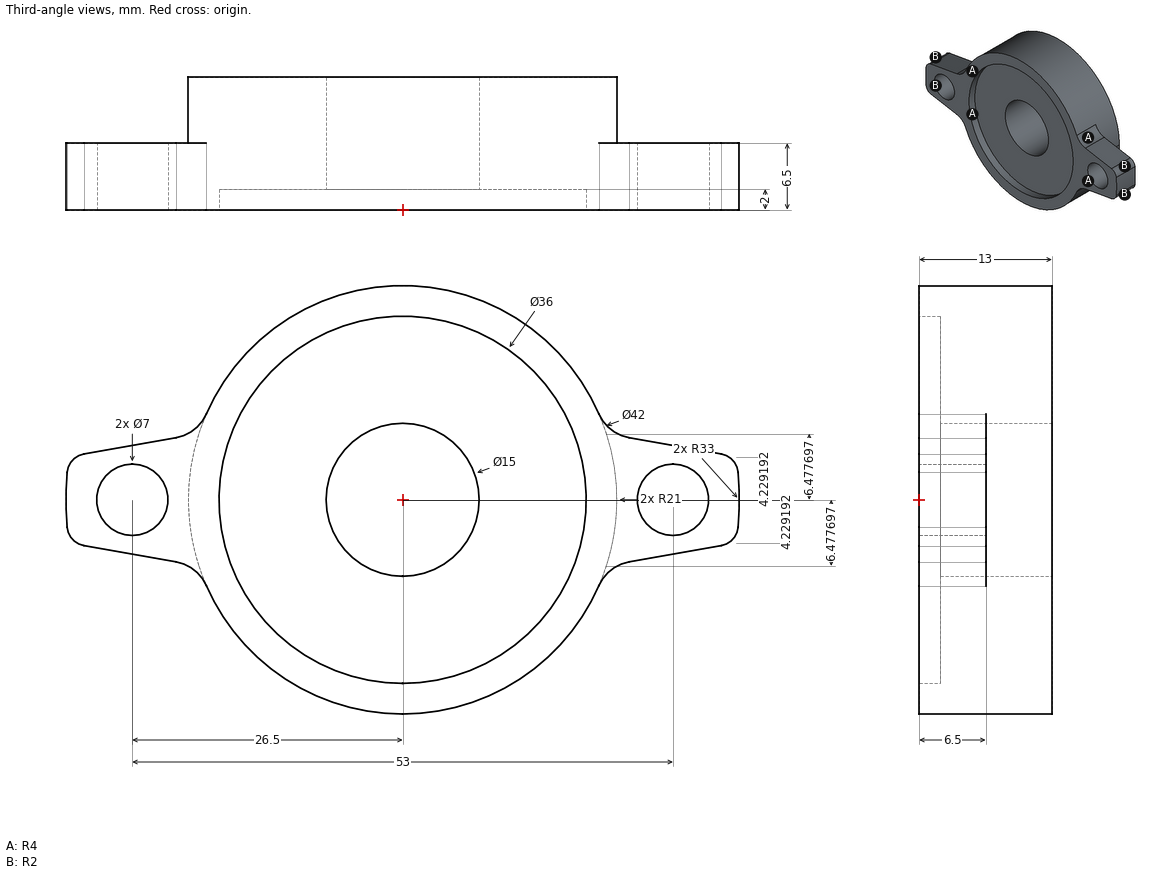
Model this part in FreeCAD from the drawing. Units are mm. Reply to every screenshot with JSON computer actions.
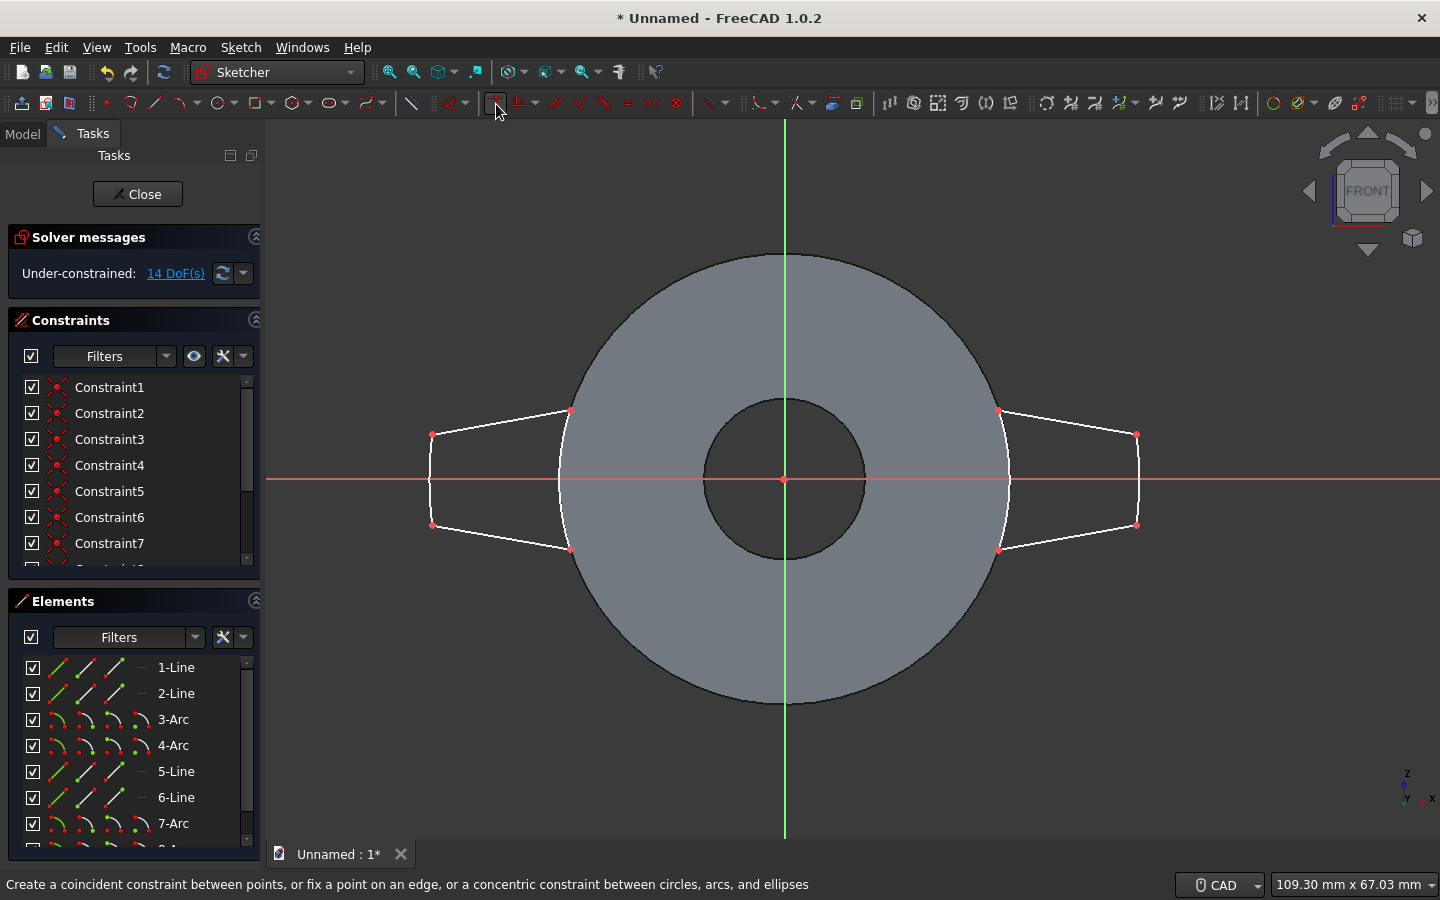
{"action": "left_click_drag", "start_coordinate": [774, 469], "coordinate": [795, 490]}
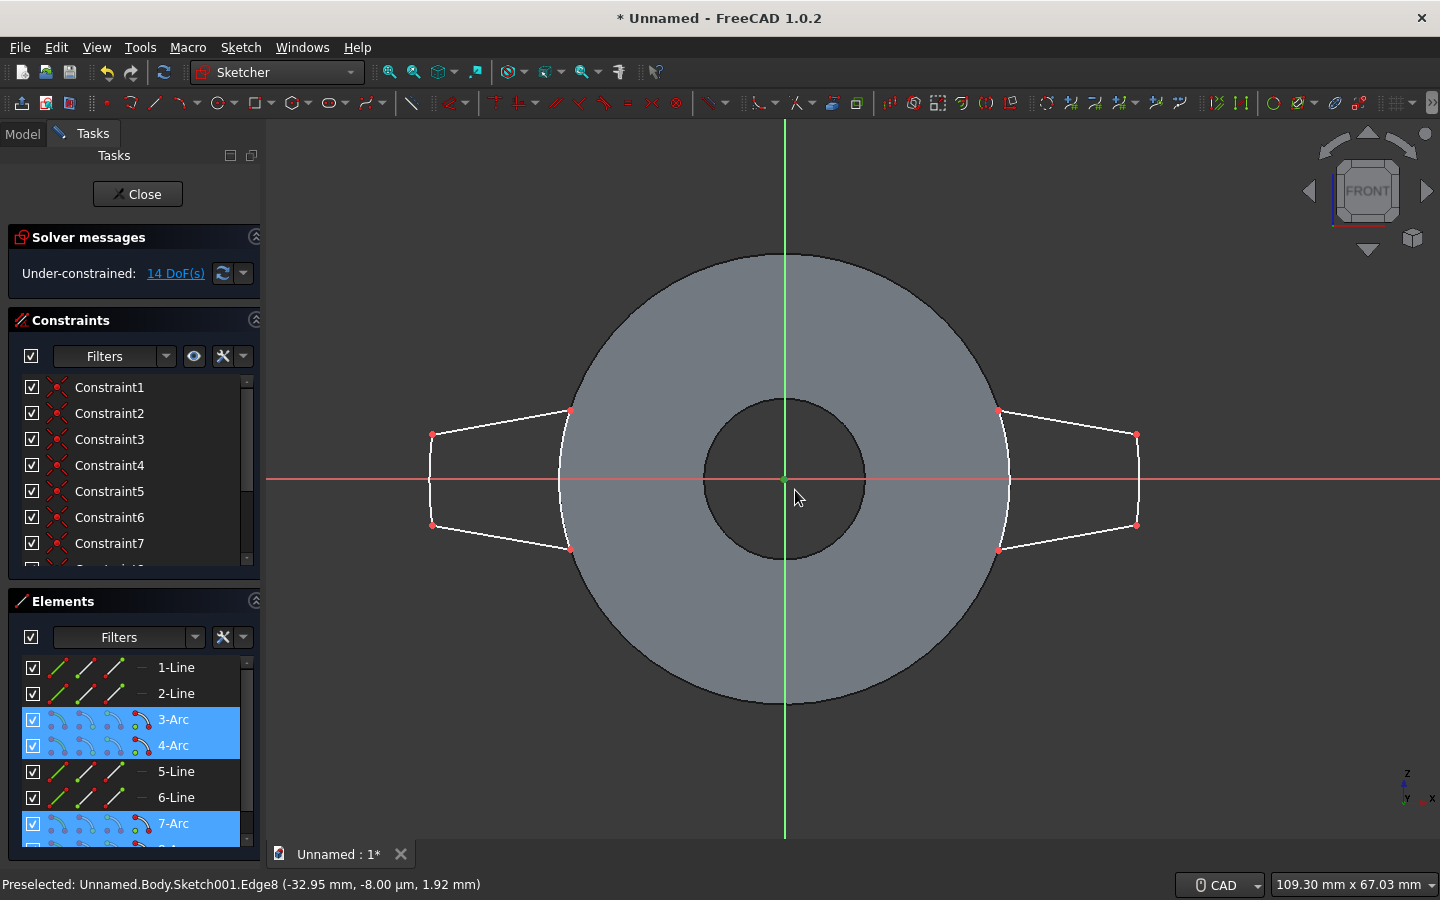
{"action": "left_click", "coordinate": [496, 104]}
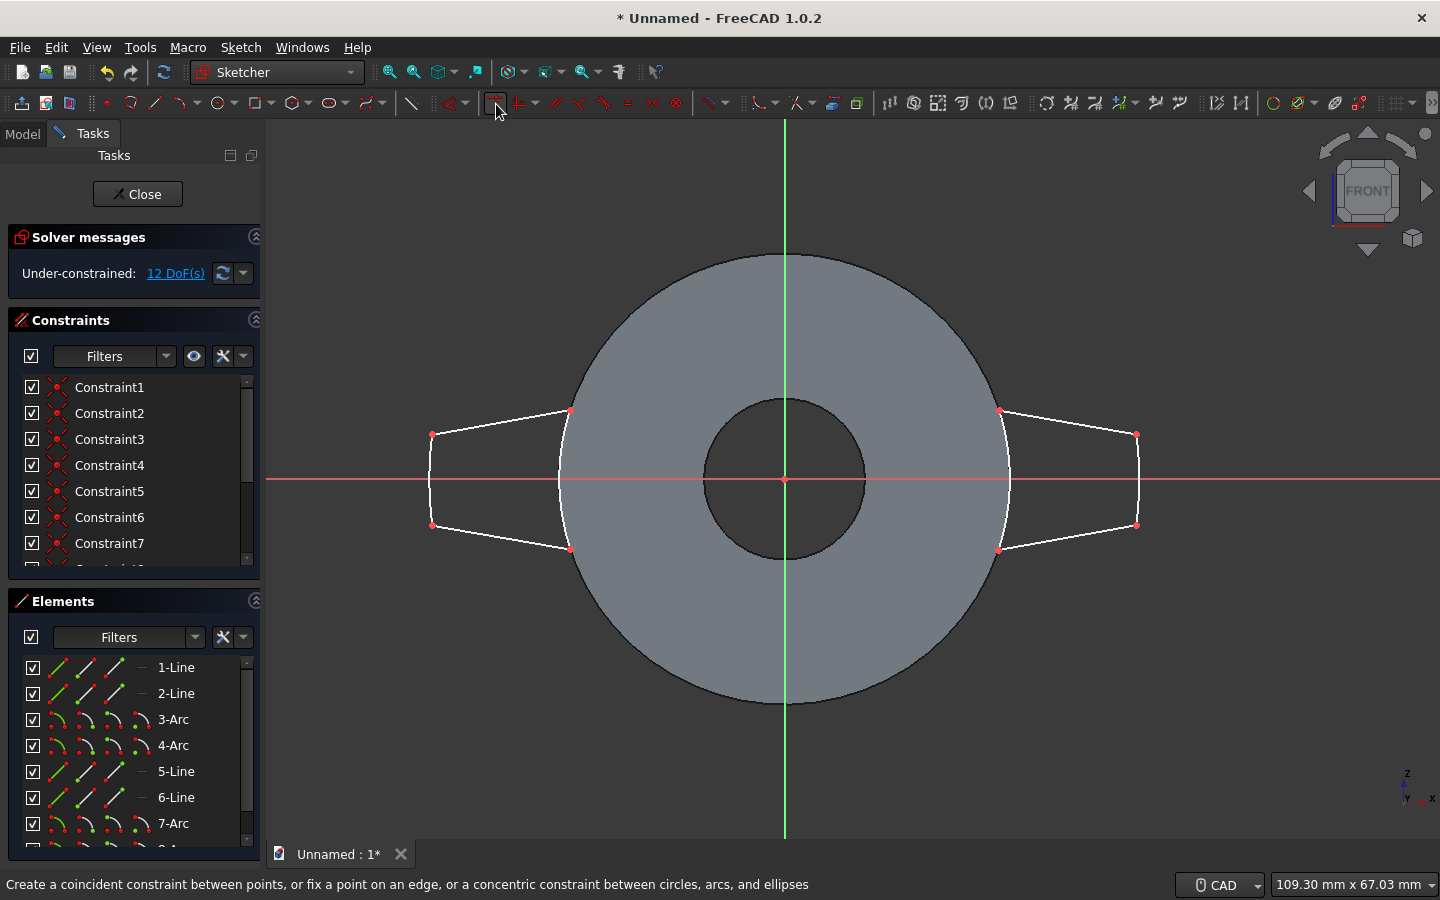
{"action": "left_click", "coordinate": [1008, 509]}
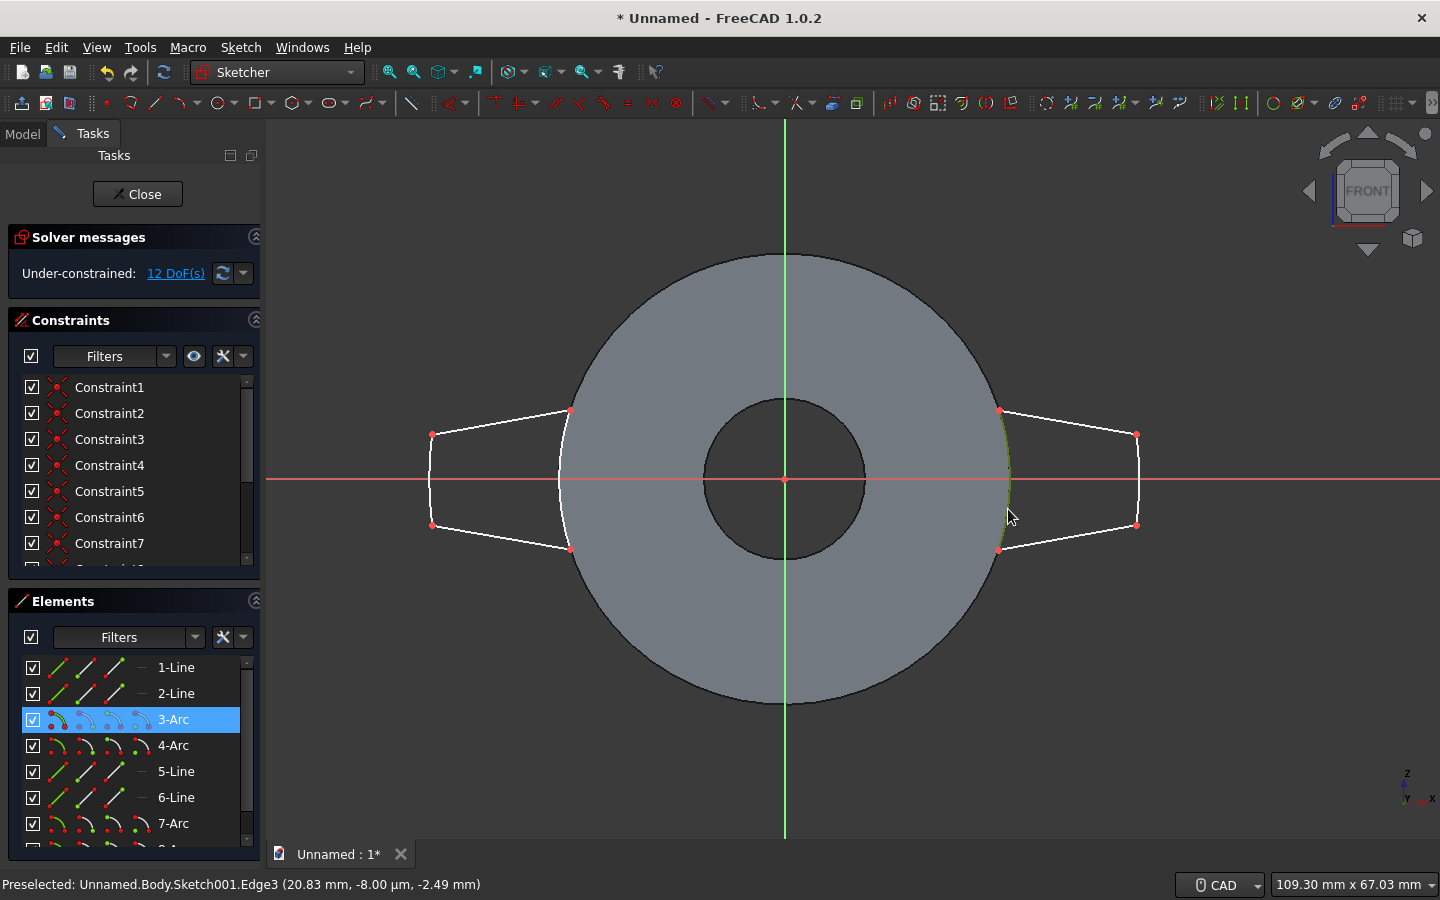
{"action": "left_click", "coordinate": [561, 452]}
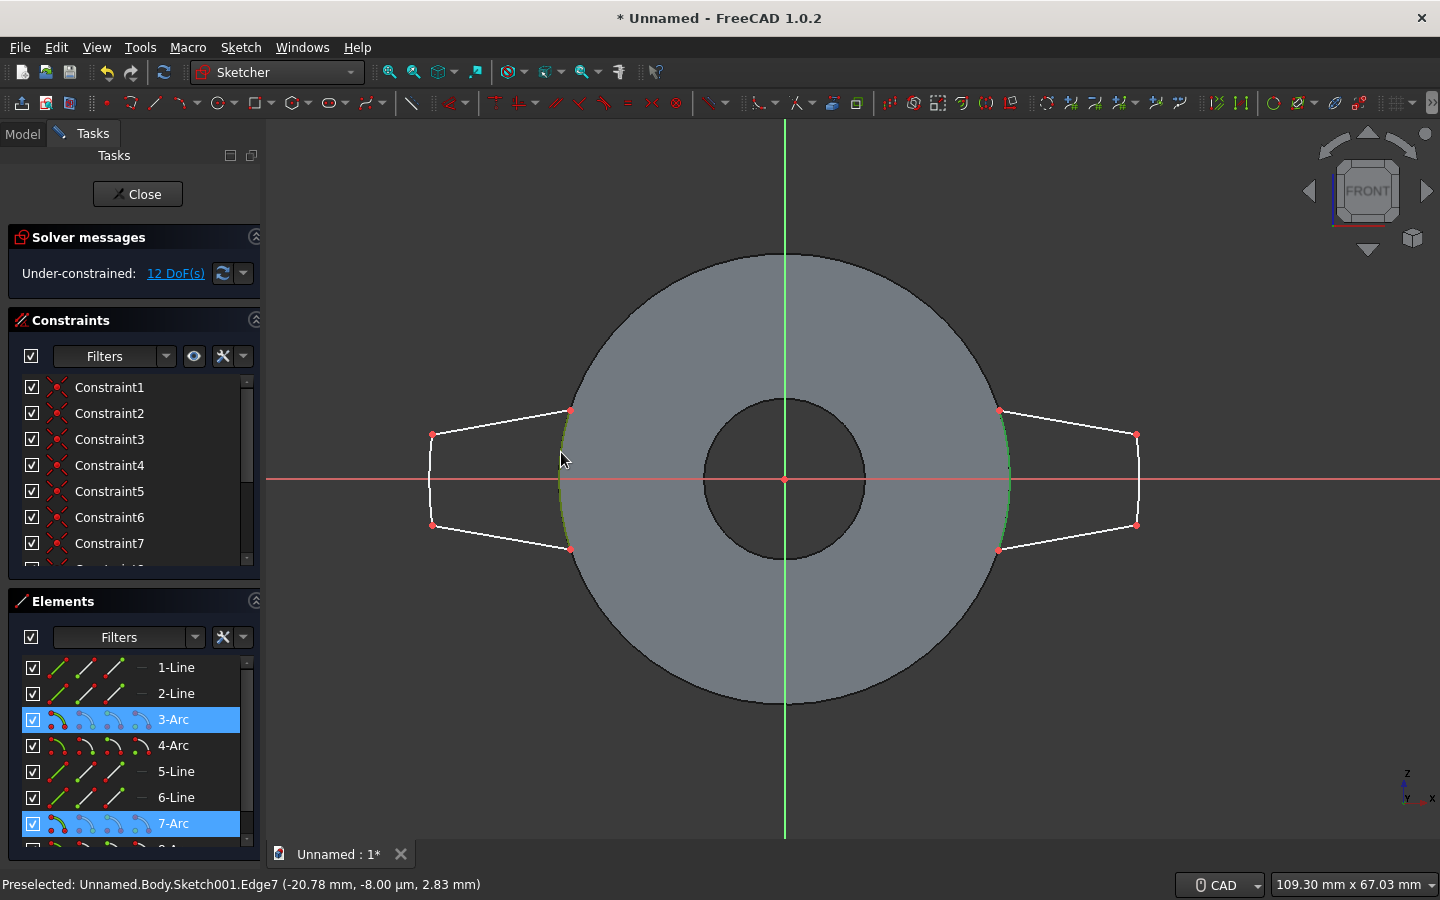
{"action": "left_click", "coordinate": [628, 104]}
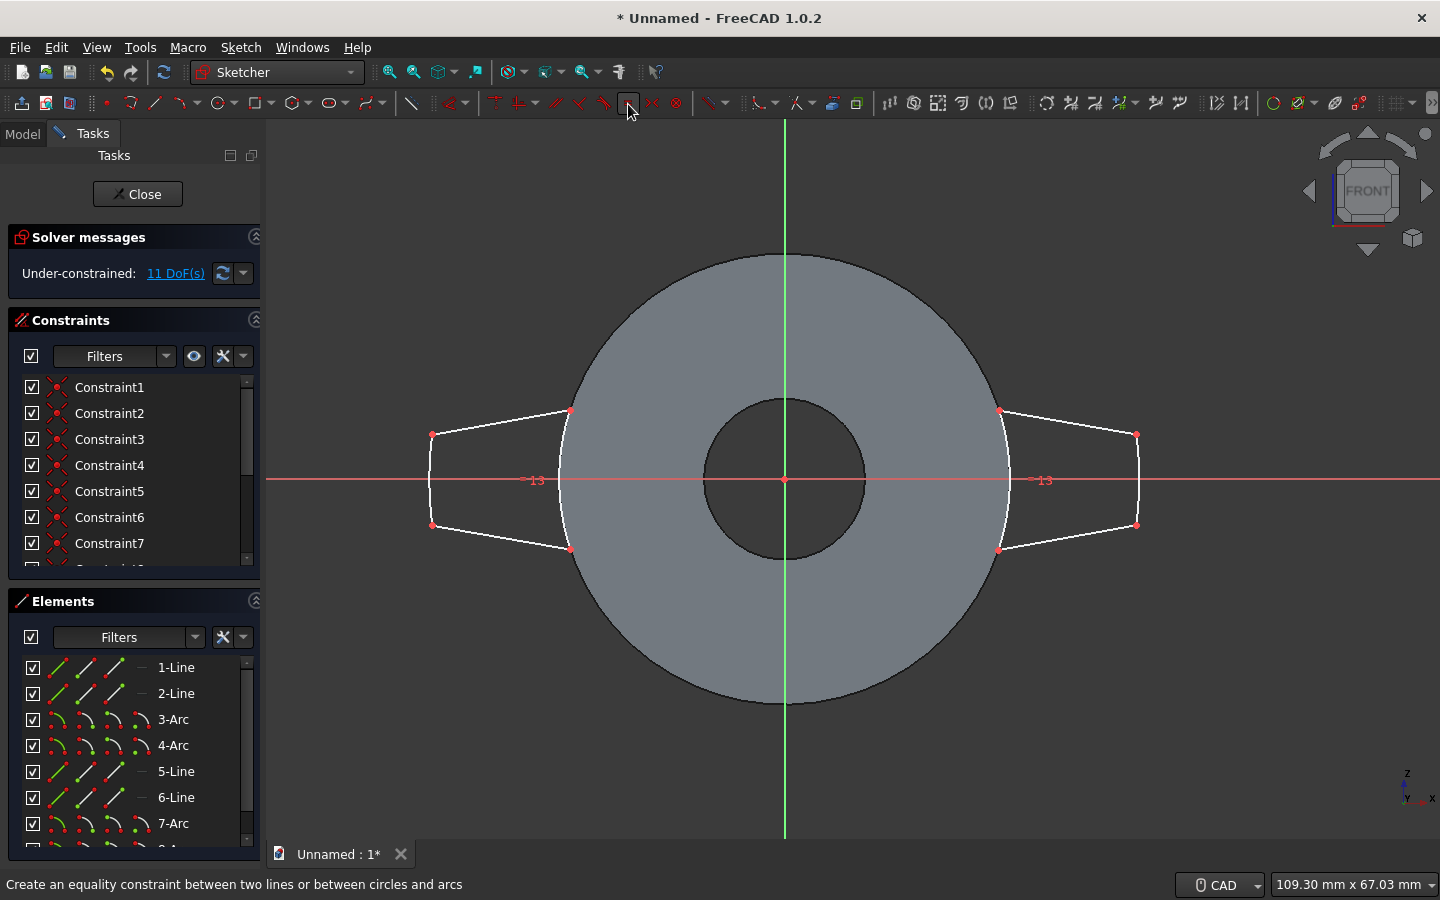
{"action": "left_click", "coordinate": [1139, 498]}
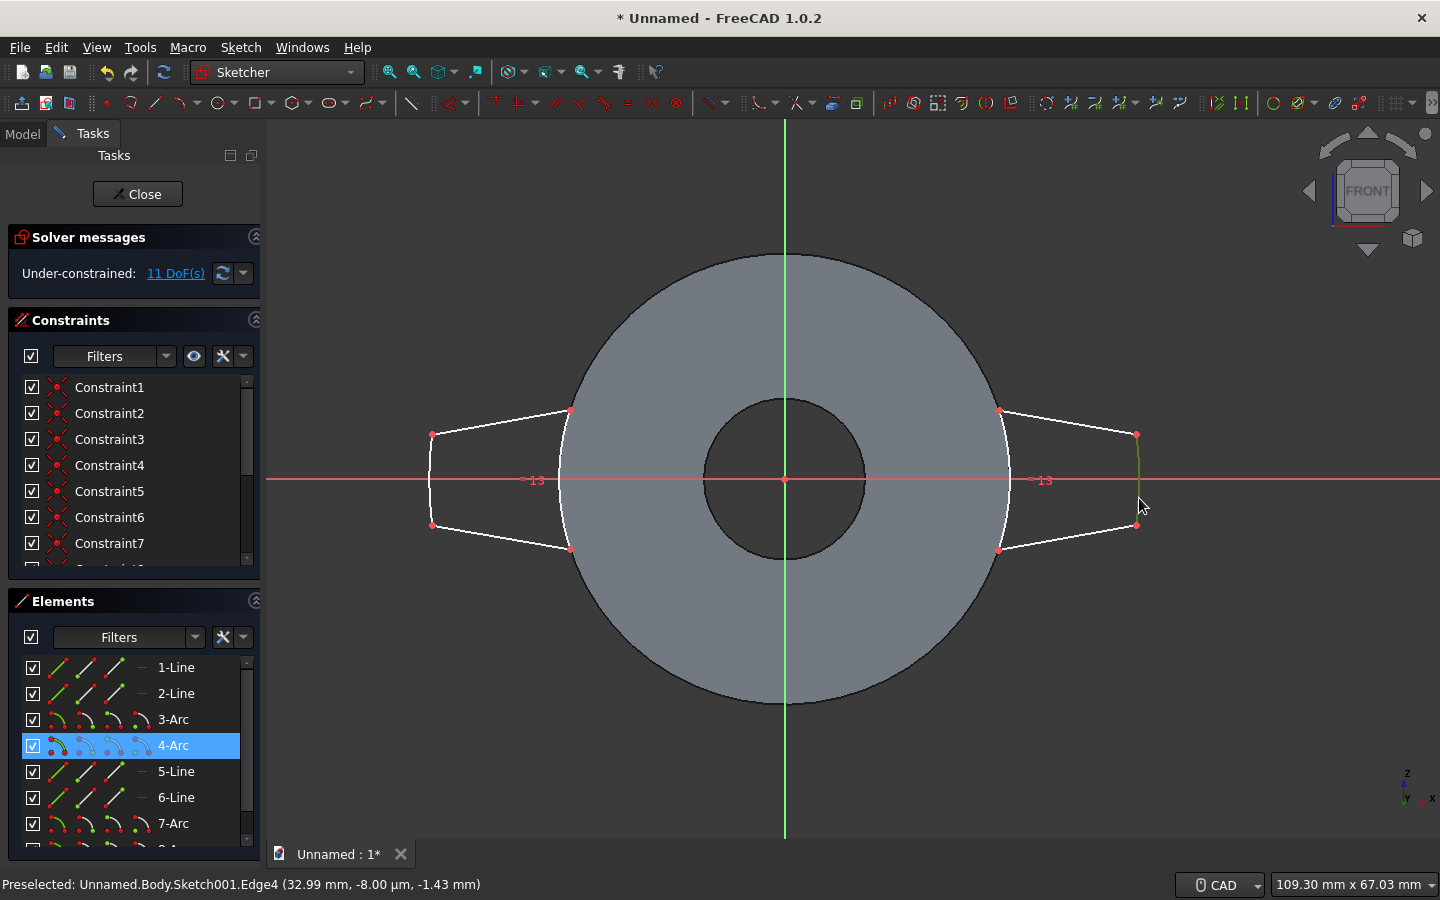
{"action": "left_click", "coordinate": [430, 462]}